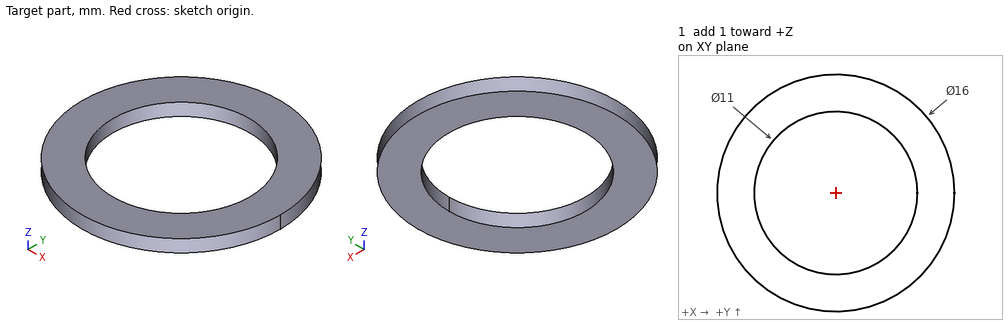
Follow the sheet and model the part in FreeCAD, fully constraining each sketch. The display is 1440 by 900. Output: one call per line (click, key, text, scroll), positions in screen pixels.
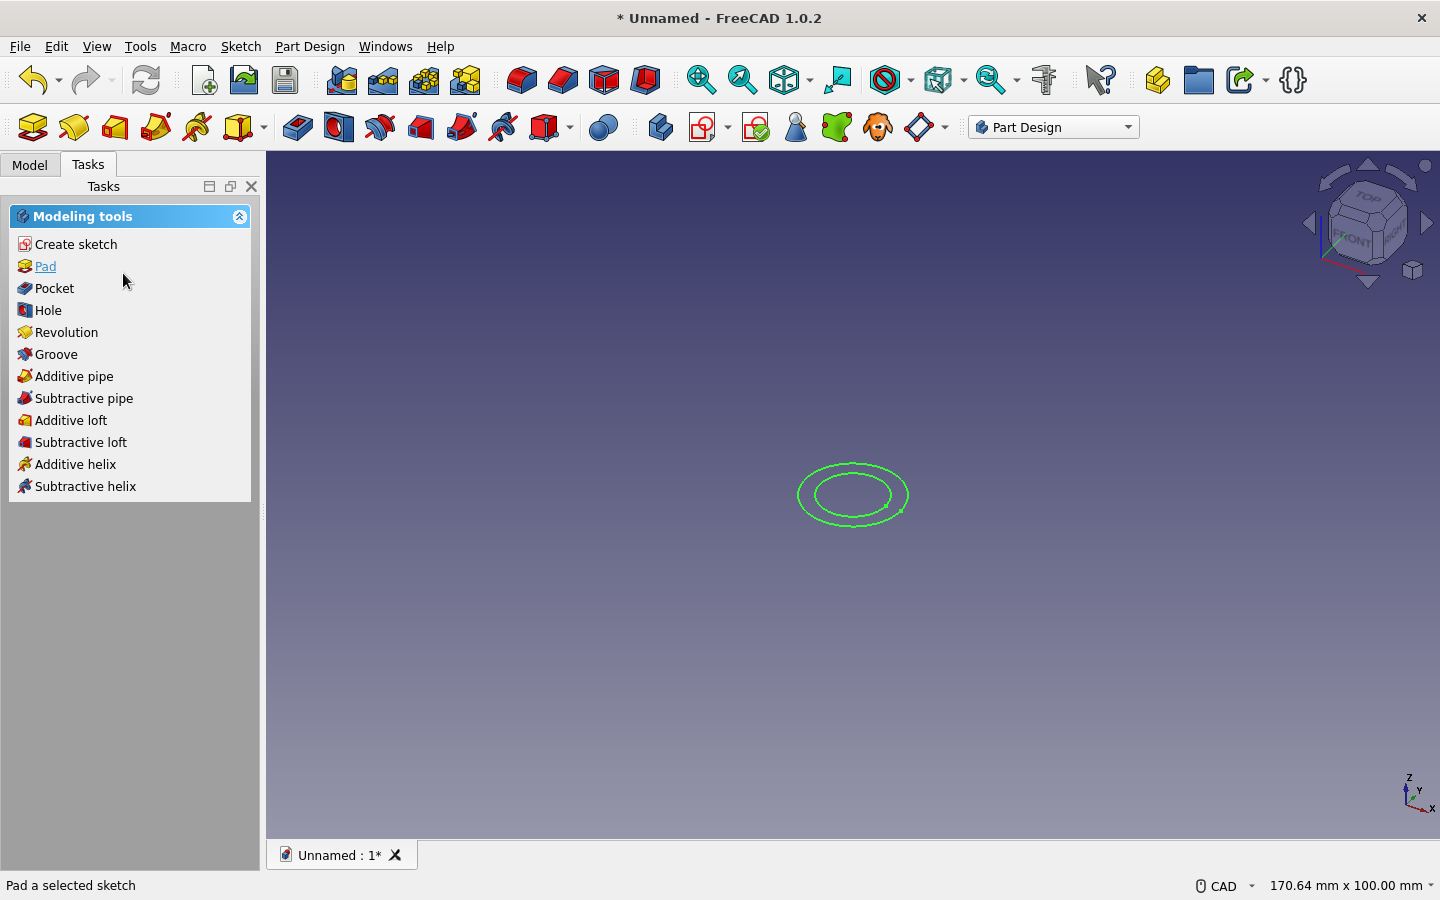
click(33, 128)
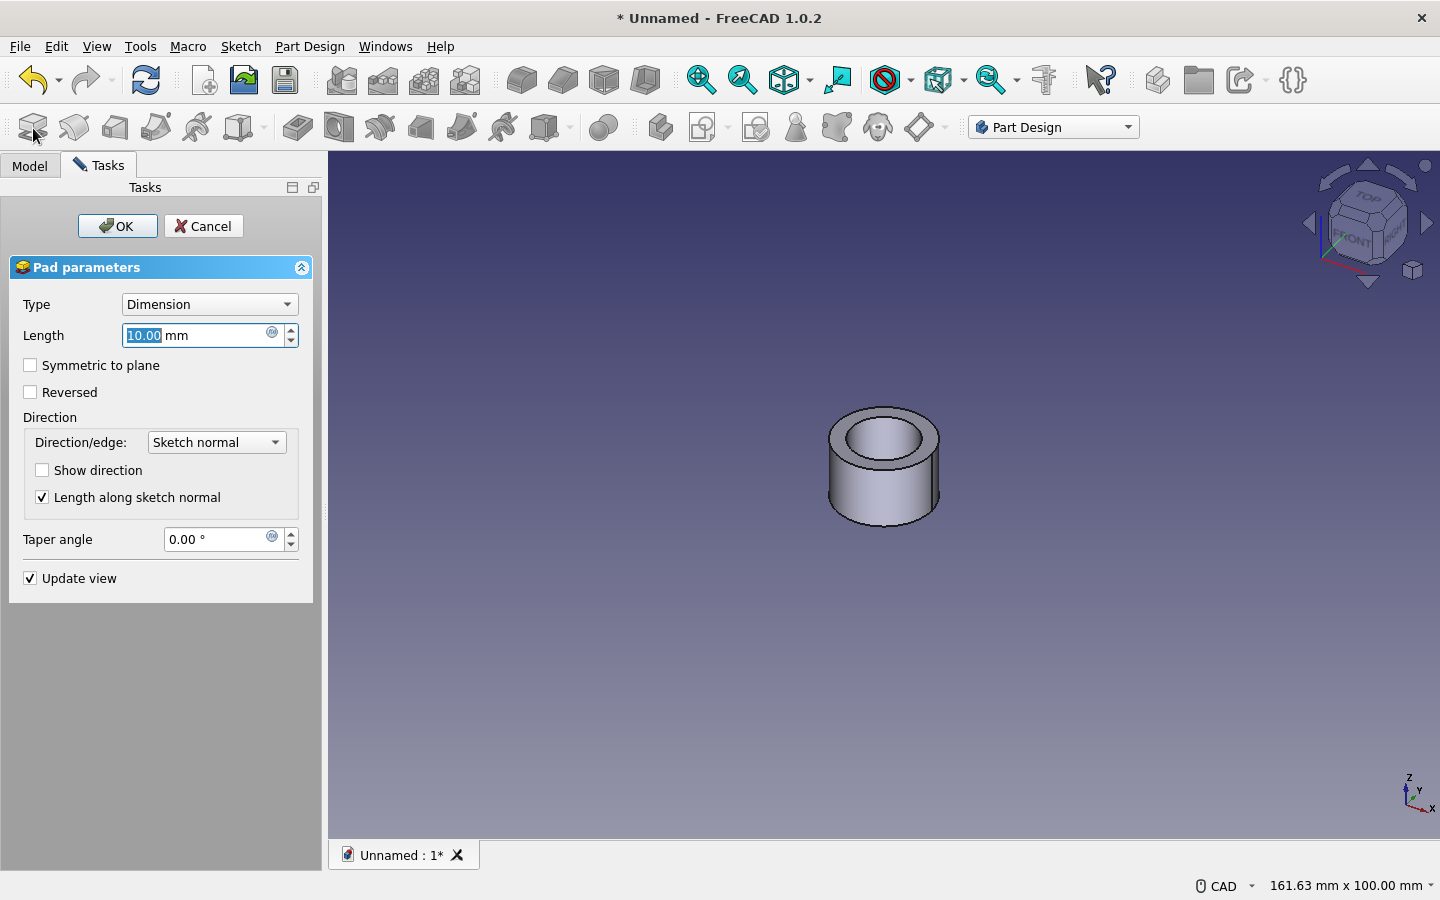
text(1)
key(Tab)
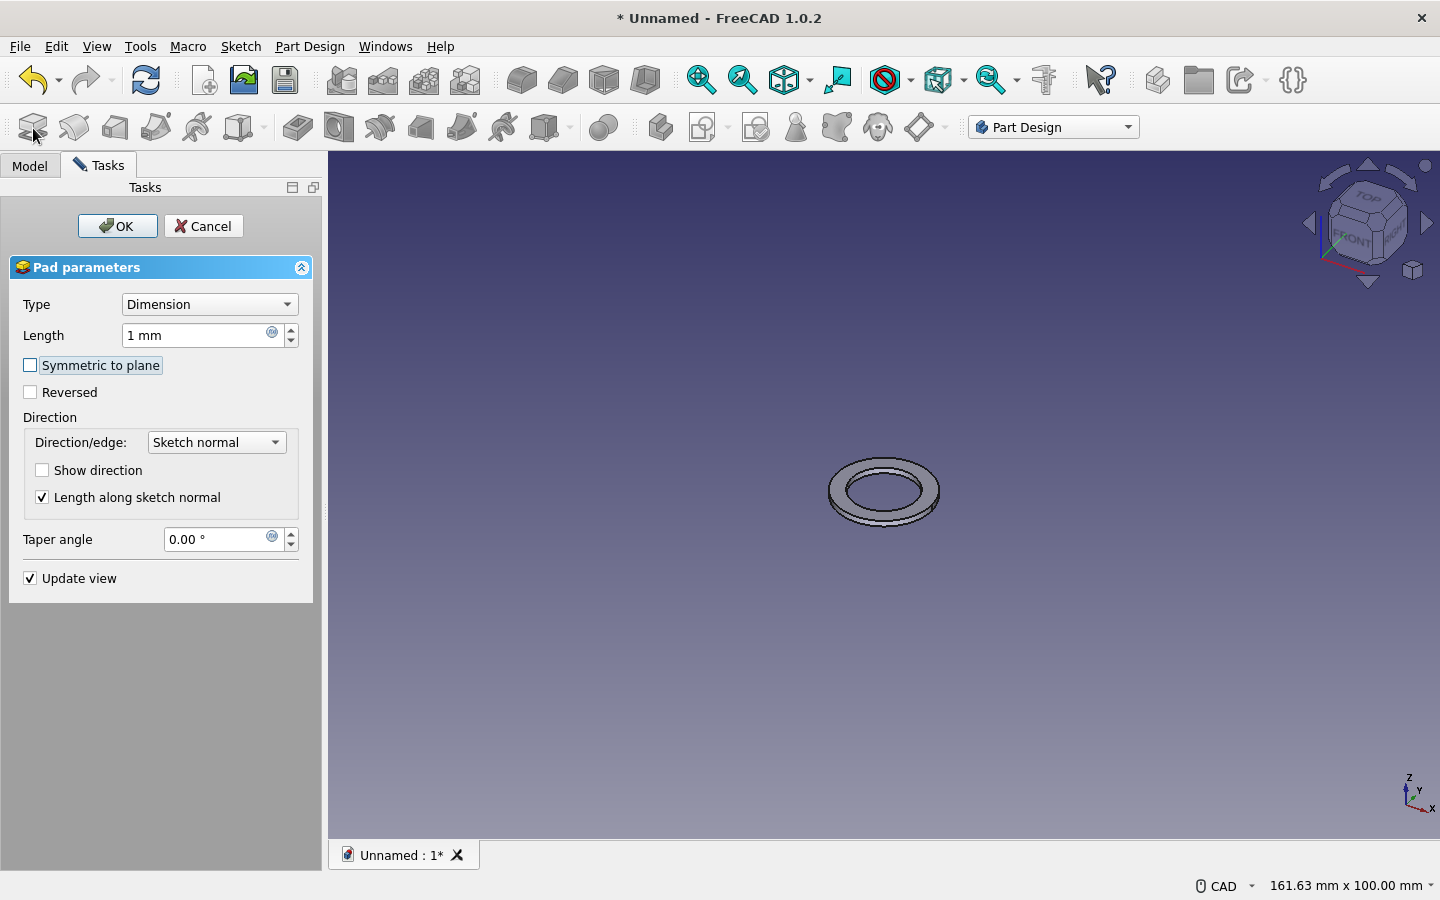
click(118, 226)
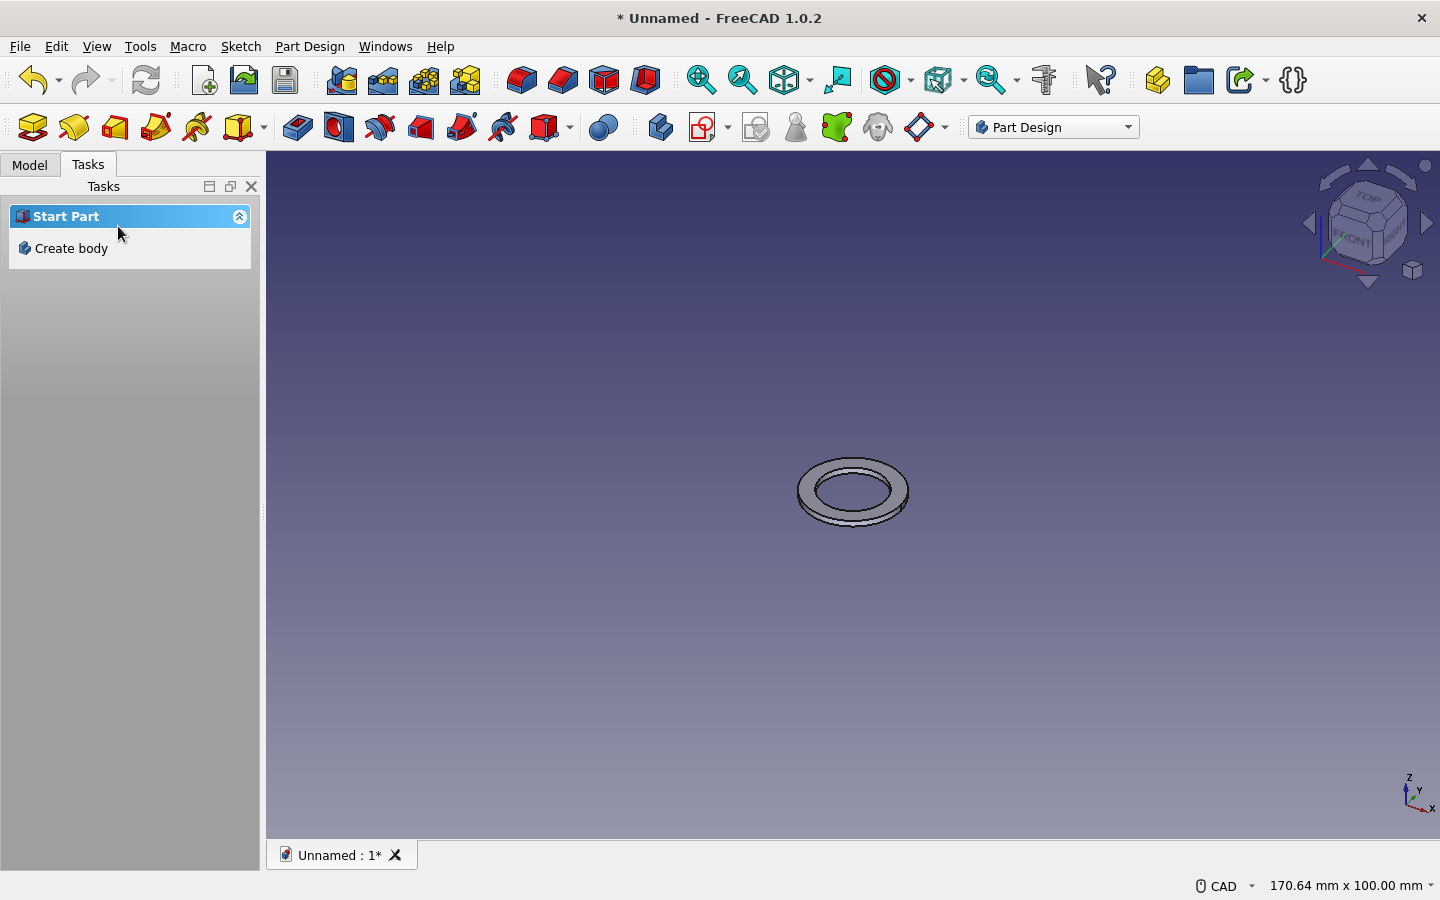
key(0)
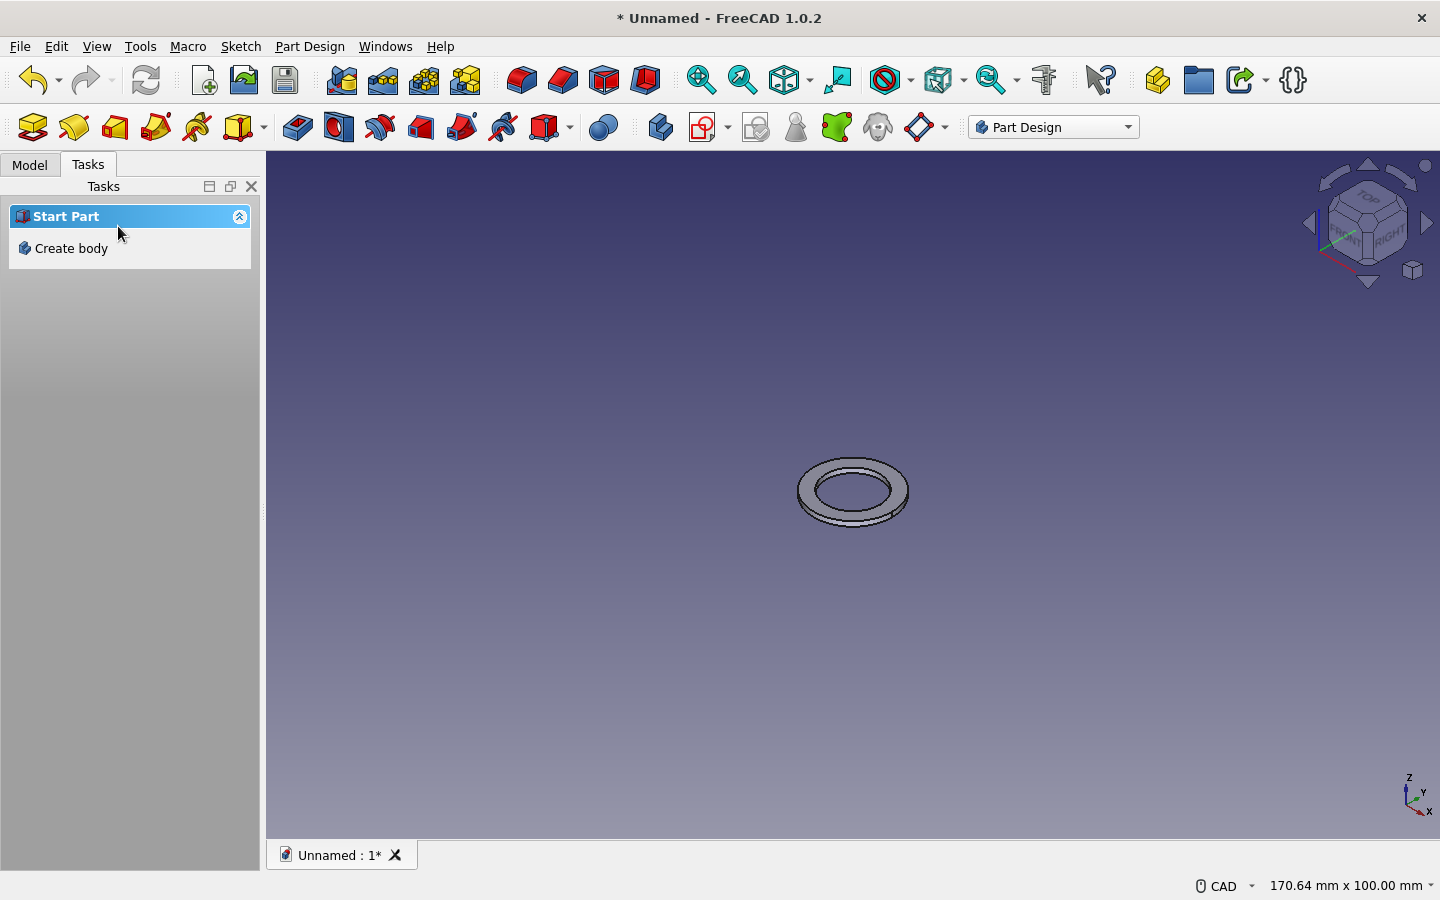
click(702, 80)